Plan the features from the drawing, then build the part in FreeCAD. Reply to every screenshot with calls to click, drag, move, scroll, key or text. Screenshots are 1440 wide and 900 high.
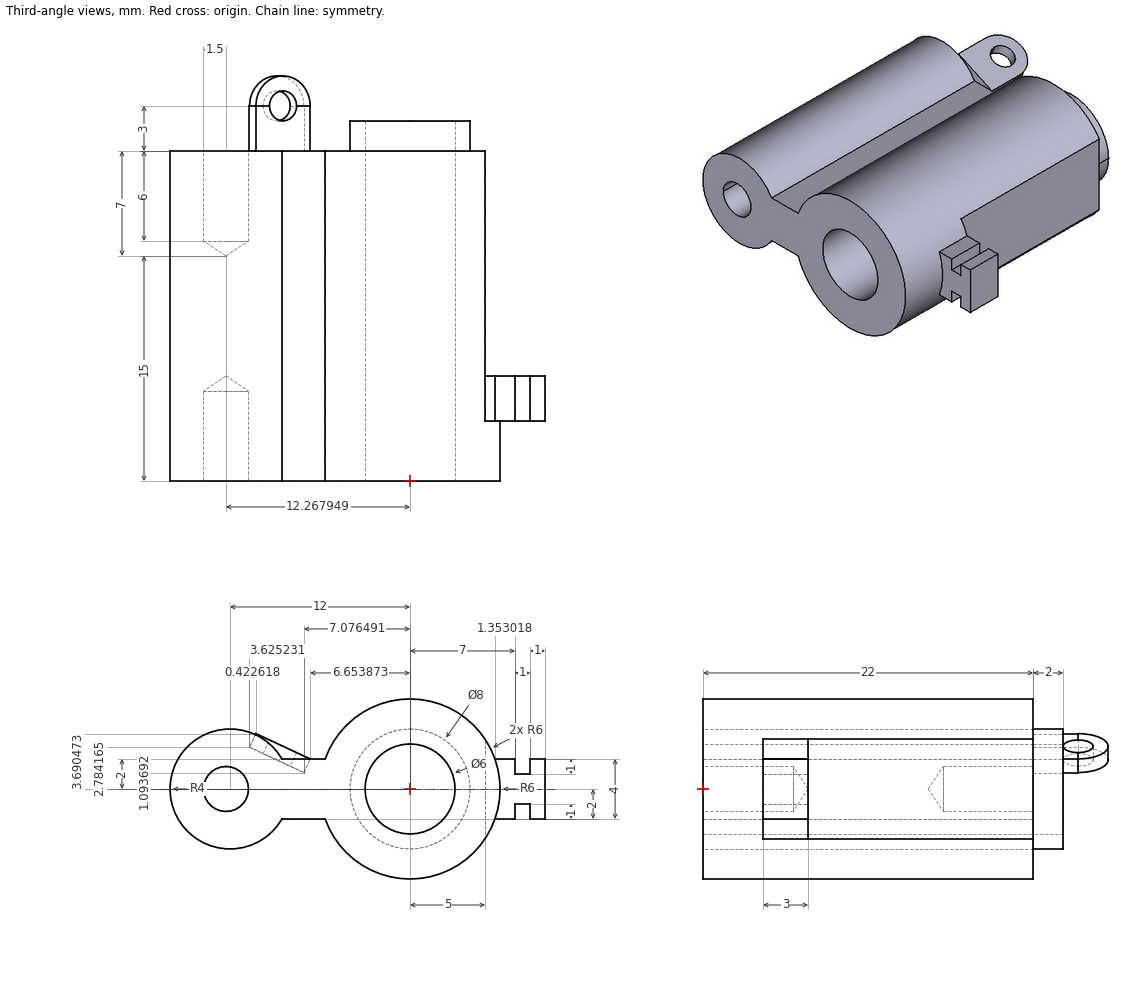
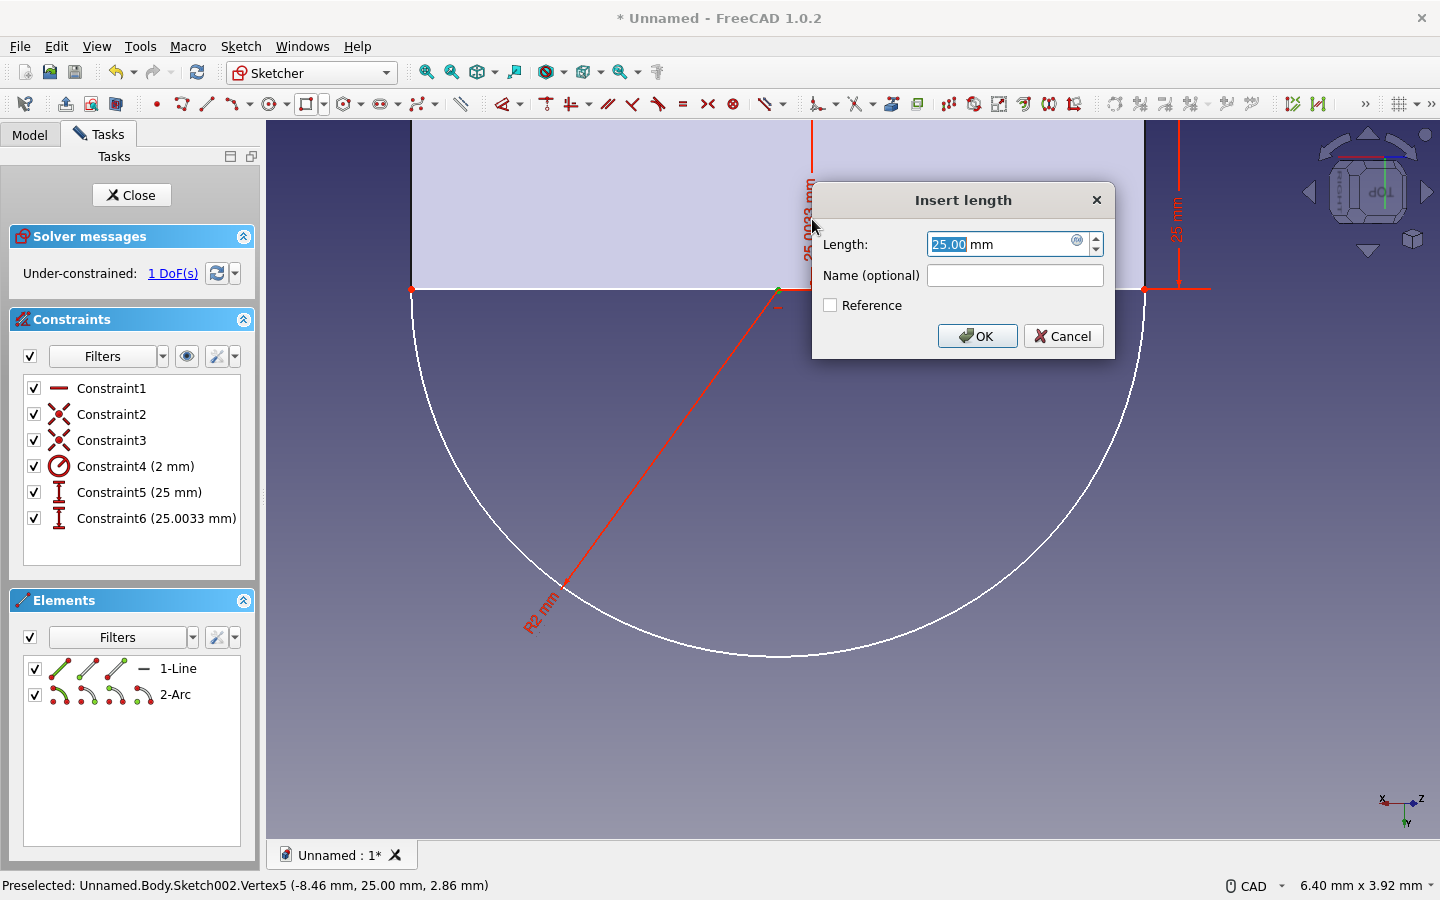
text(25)
key(Return)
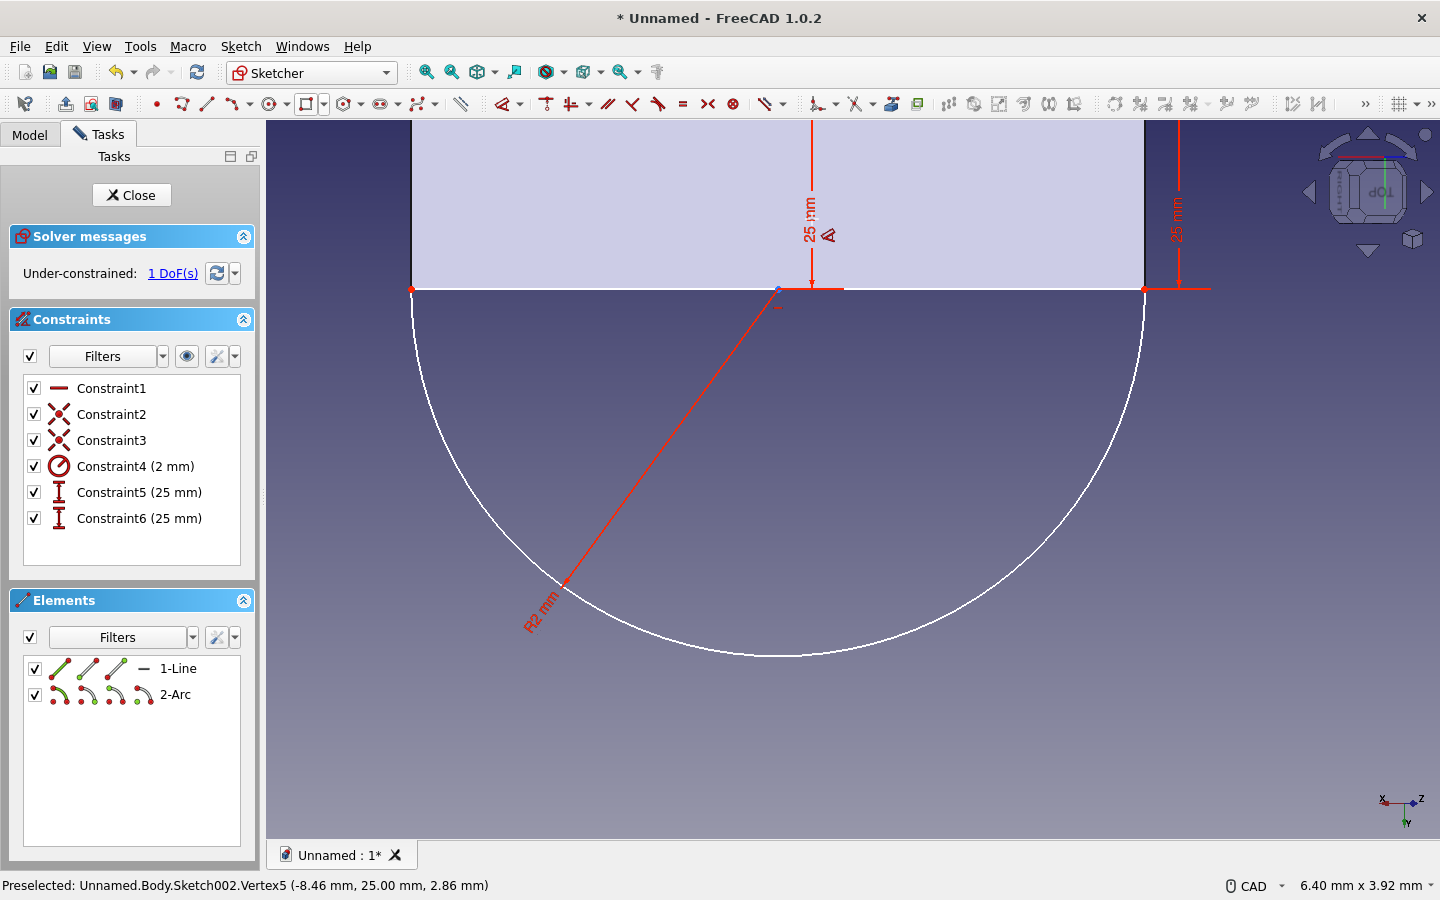
click(411, 289)
click(353, 323)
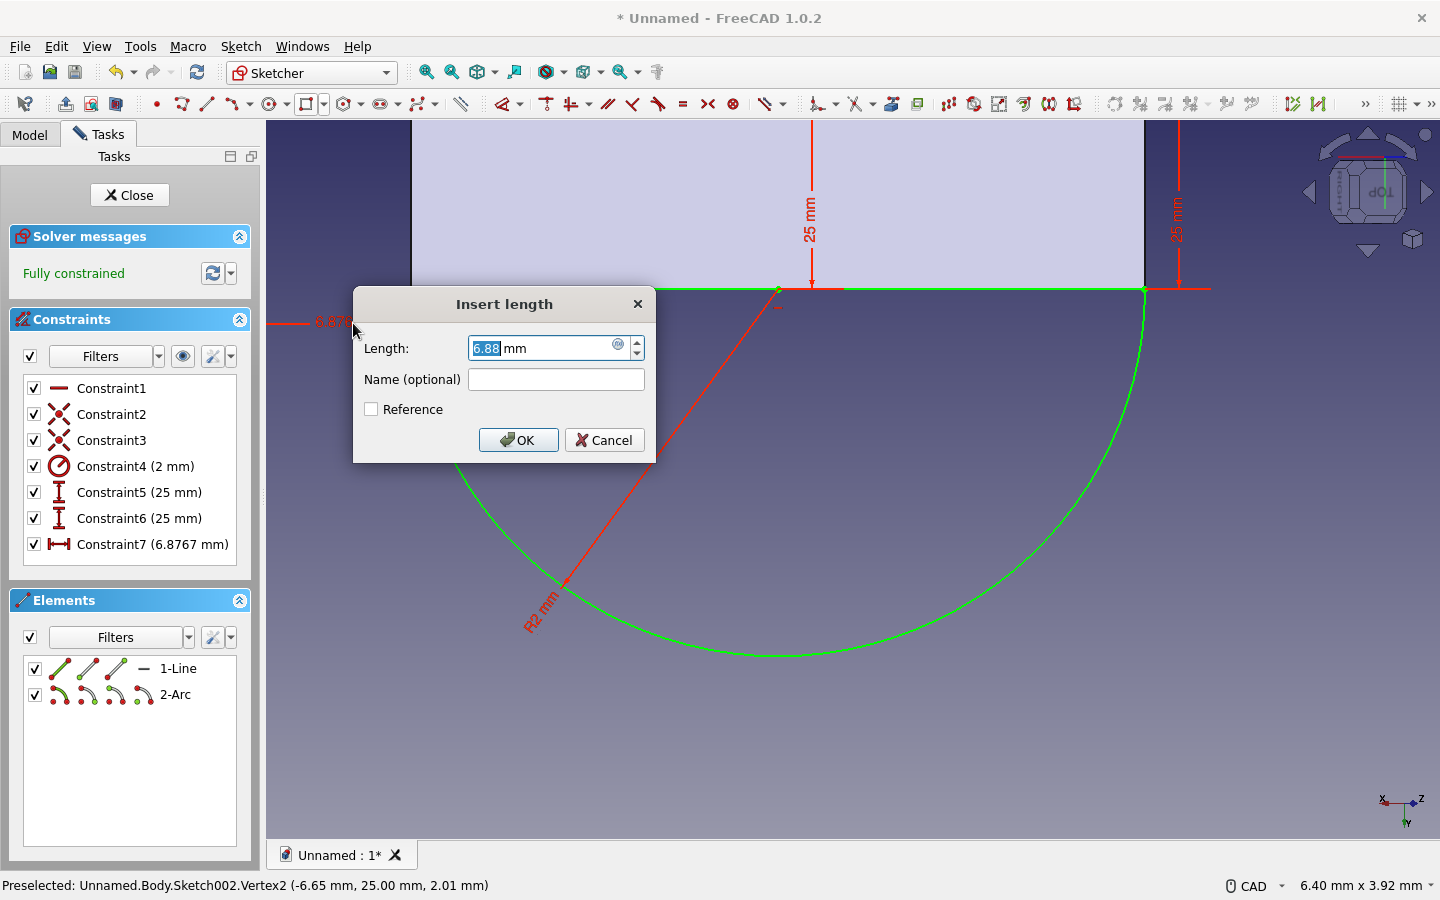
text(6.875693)
key(Return)
key(Escape)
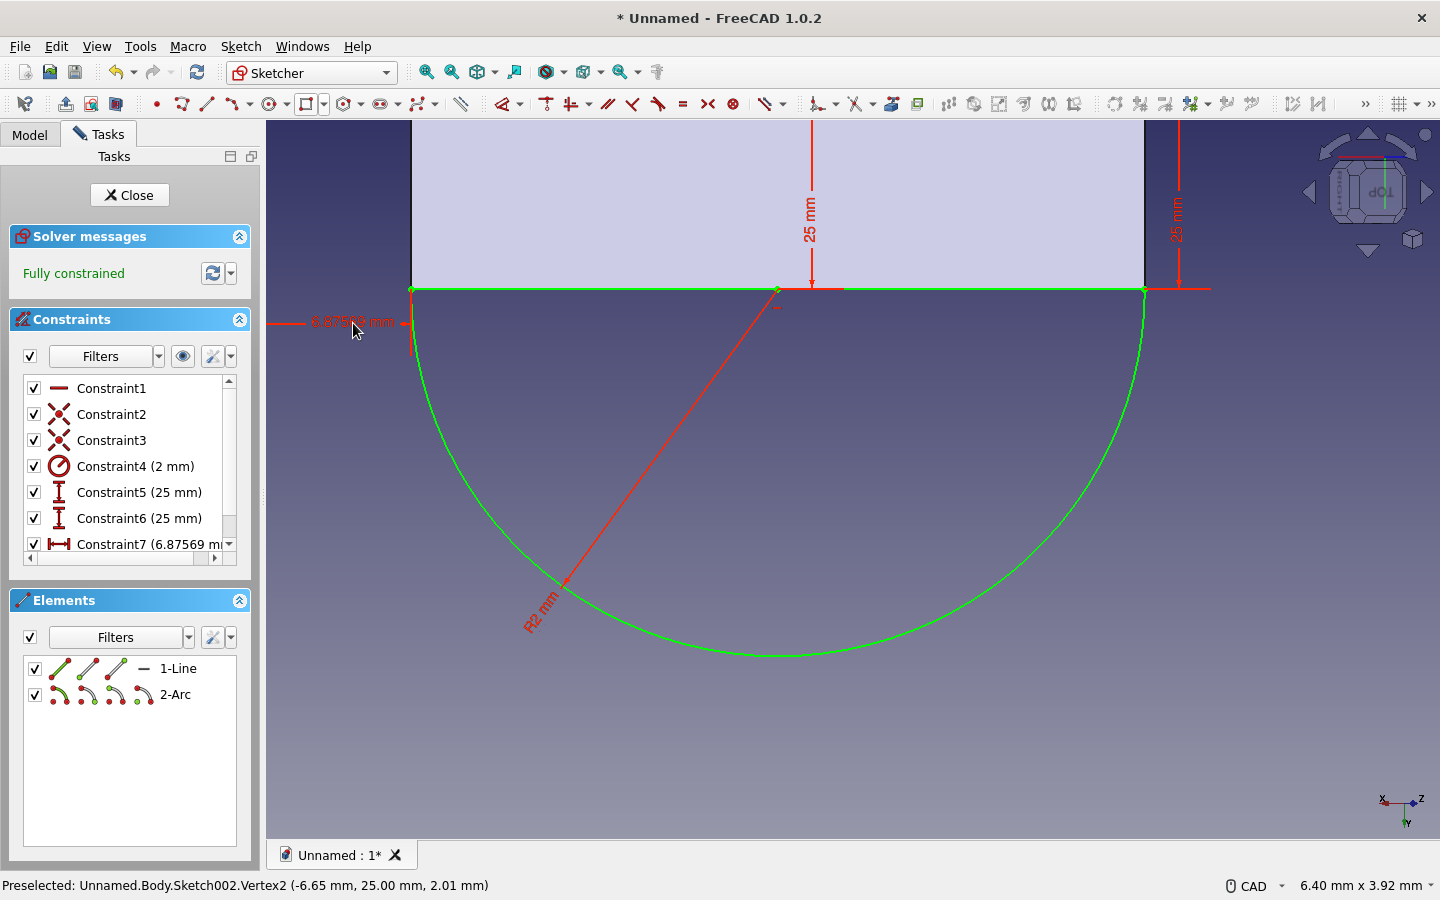
click(130, 195)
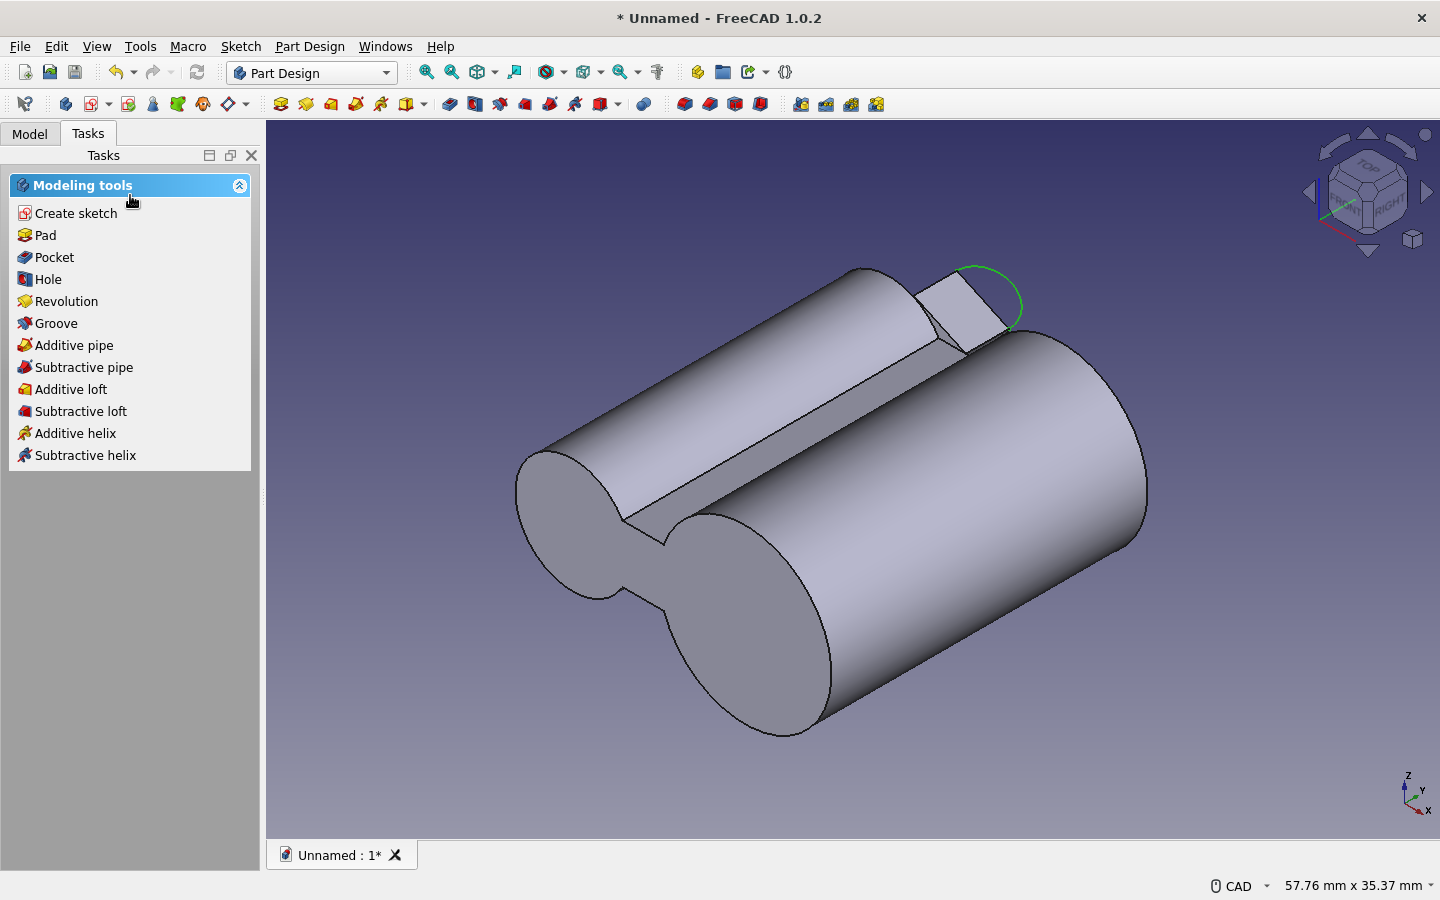
click(281, 104)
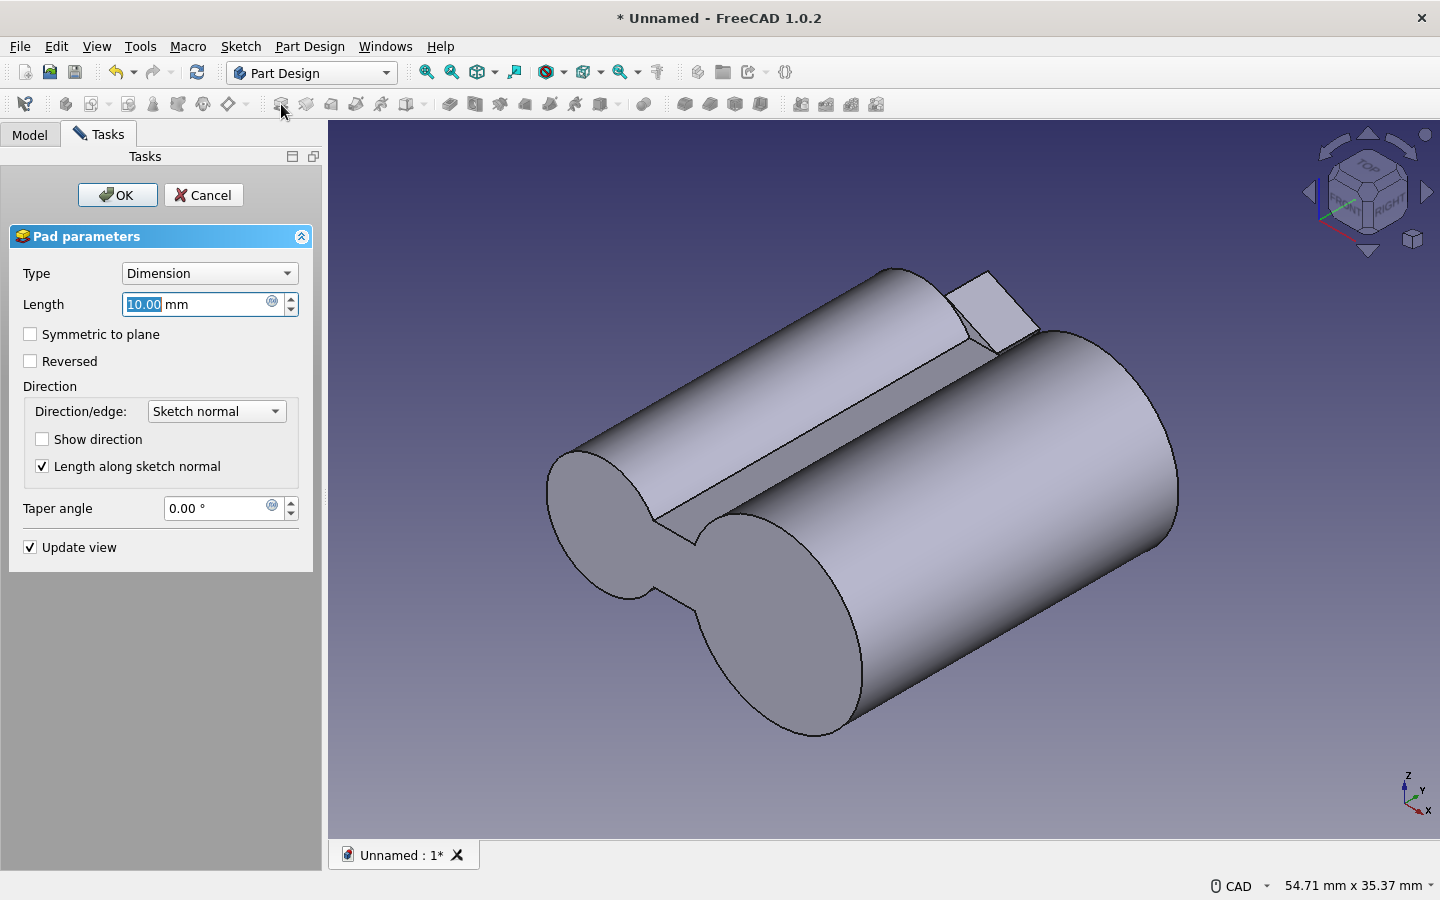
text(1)
key(Tab)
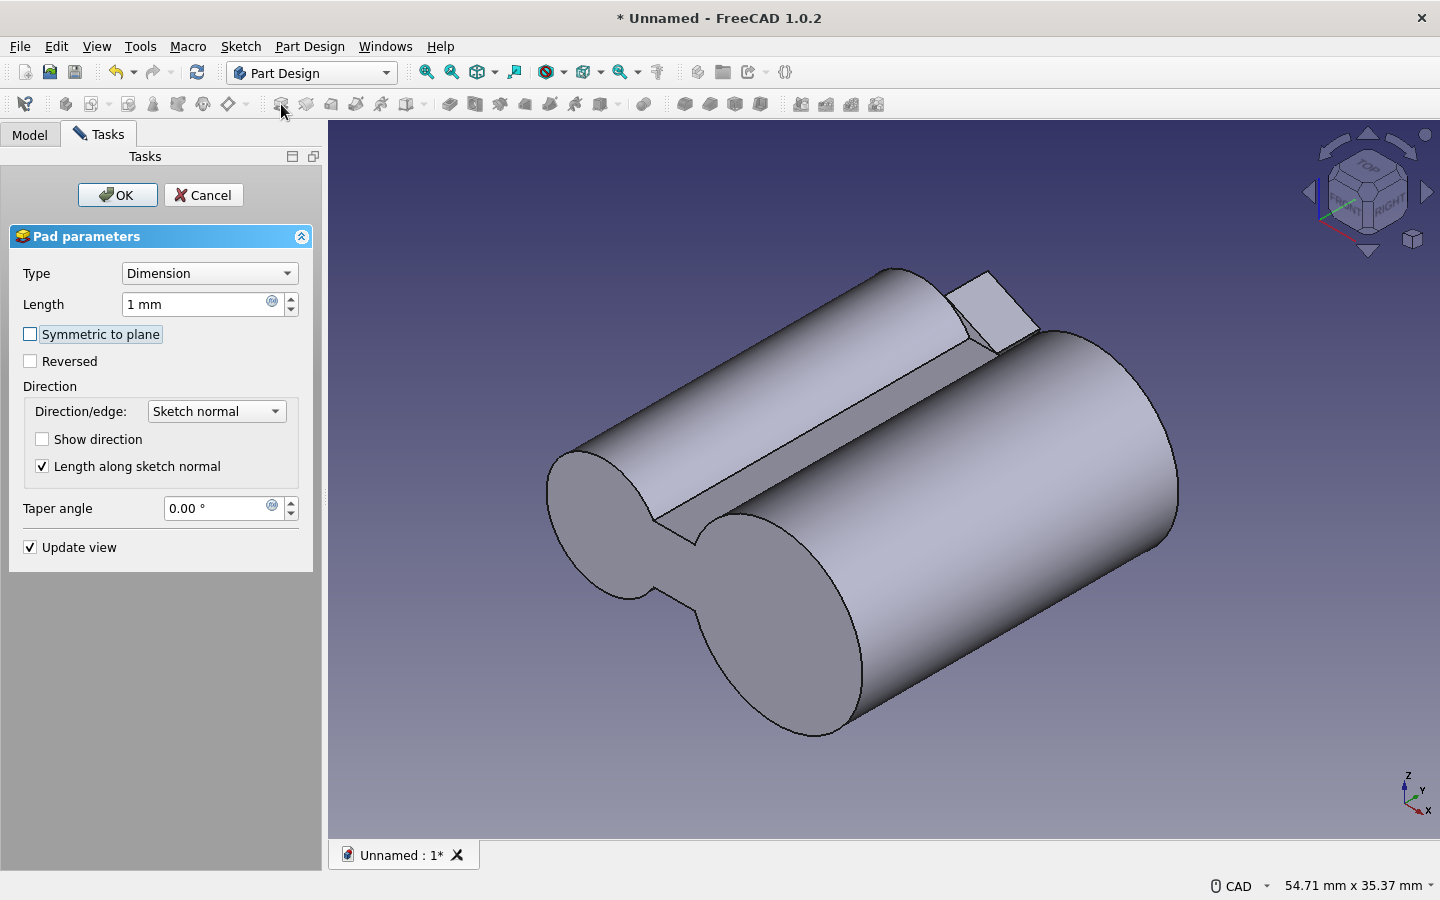
click(31, 361)